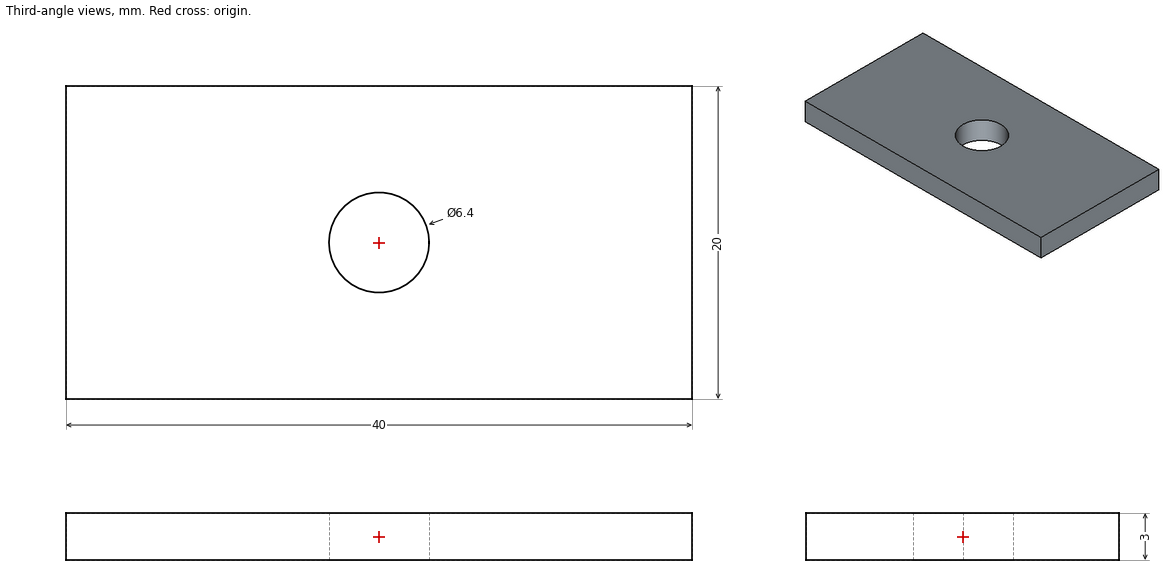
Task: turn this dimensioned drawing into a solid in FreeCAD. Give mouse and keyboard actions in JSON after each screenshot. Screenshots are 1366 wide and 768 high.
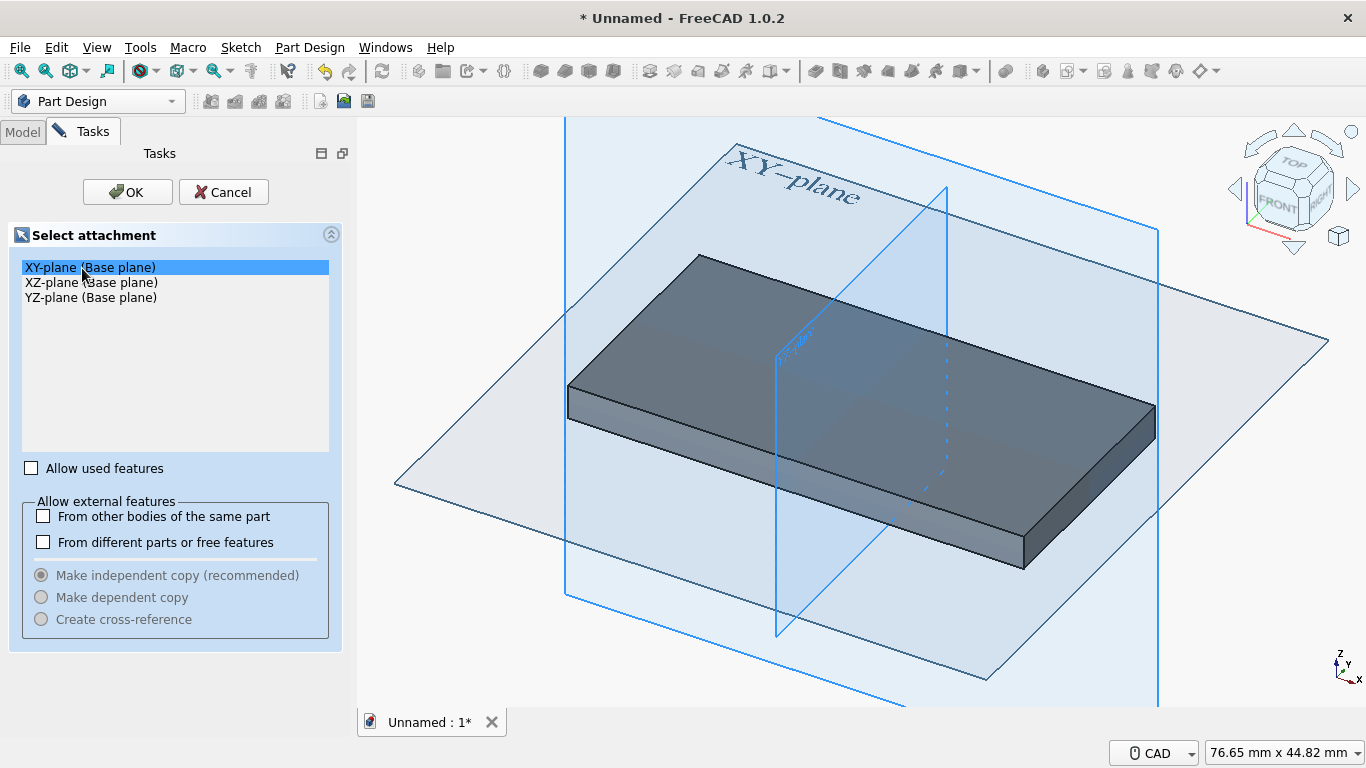
{"action": "left_click", "coordinate": [128, 192]}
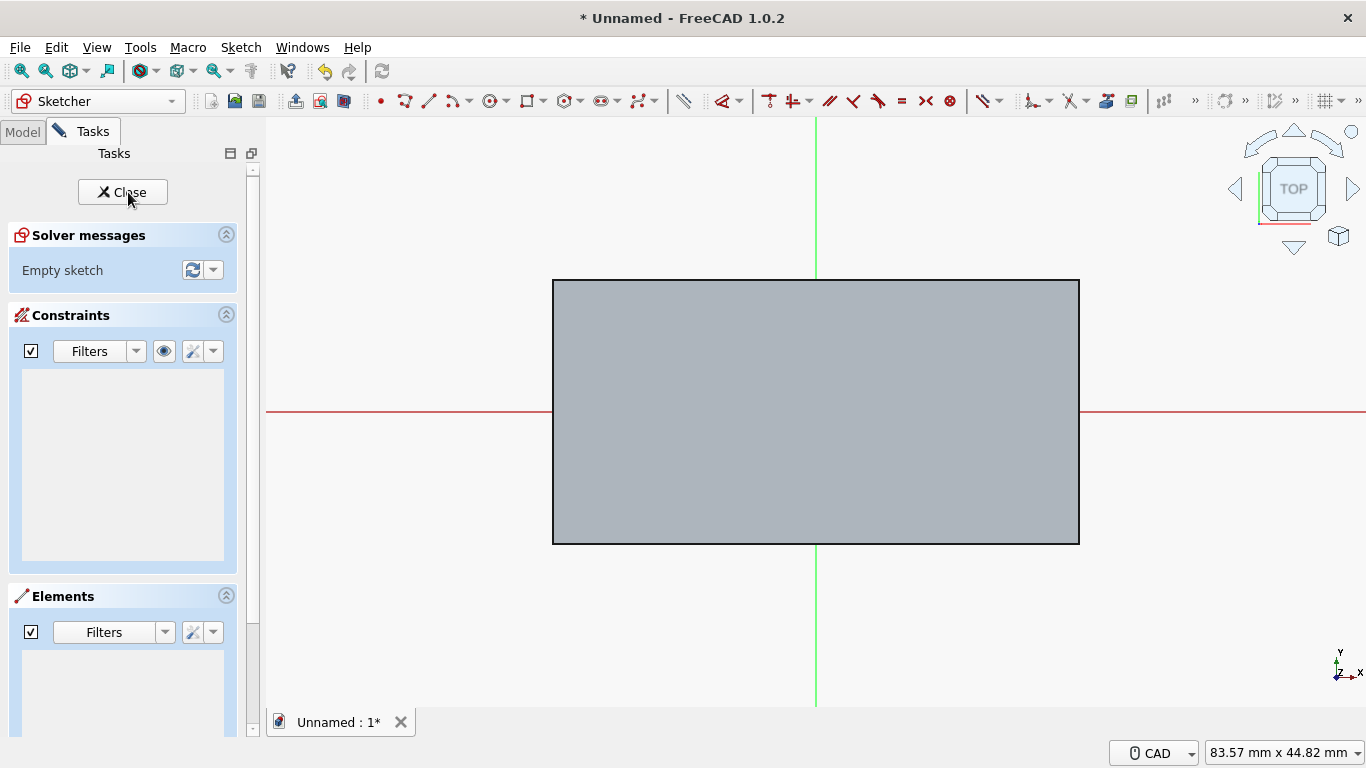
{"action": "key", "text": "q s"}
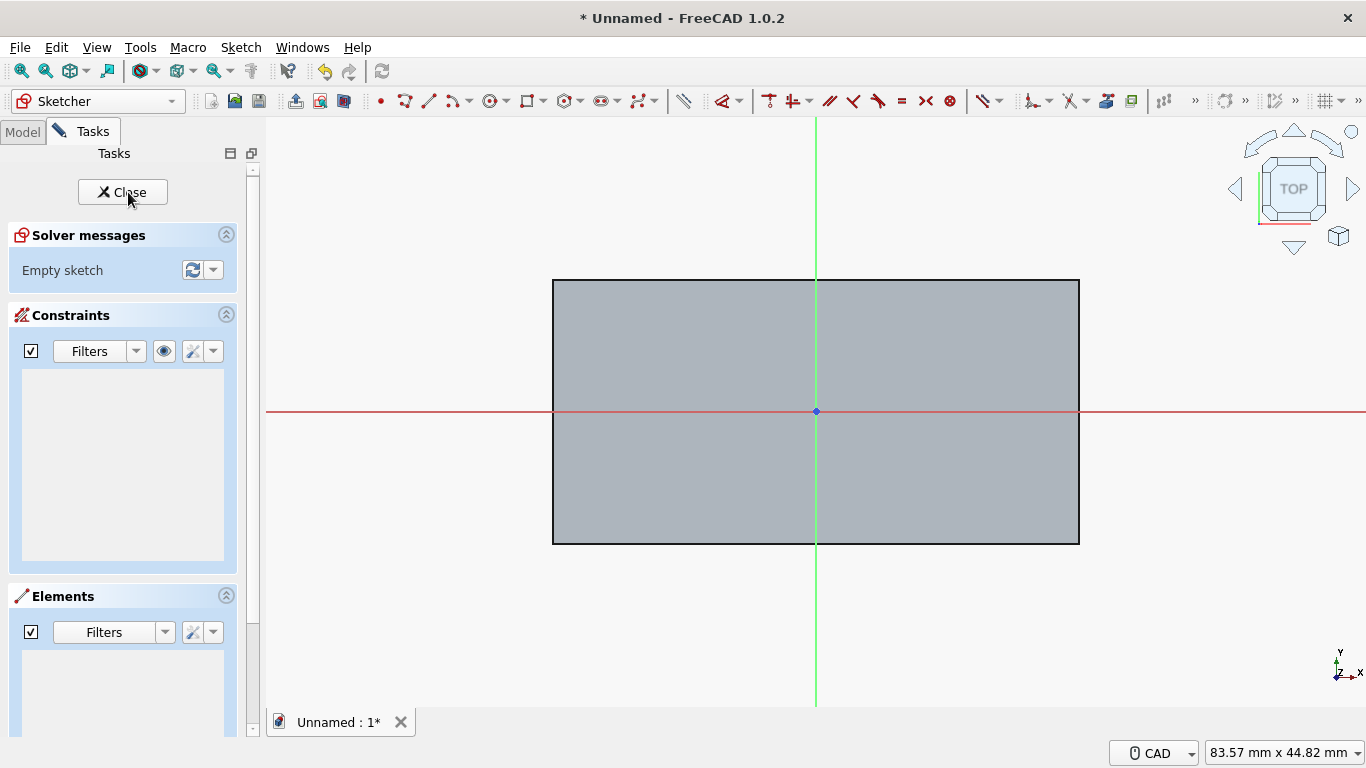
{"action": "scroll", "coordinate": [838, 412], "scroll_direction": "up", "scroll_amount": 7}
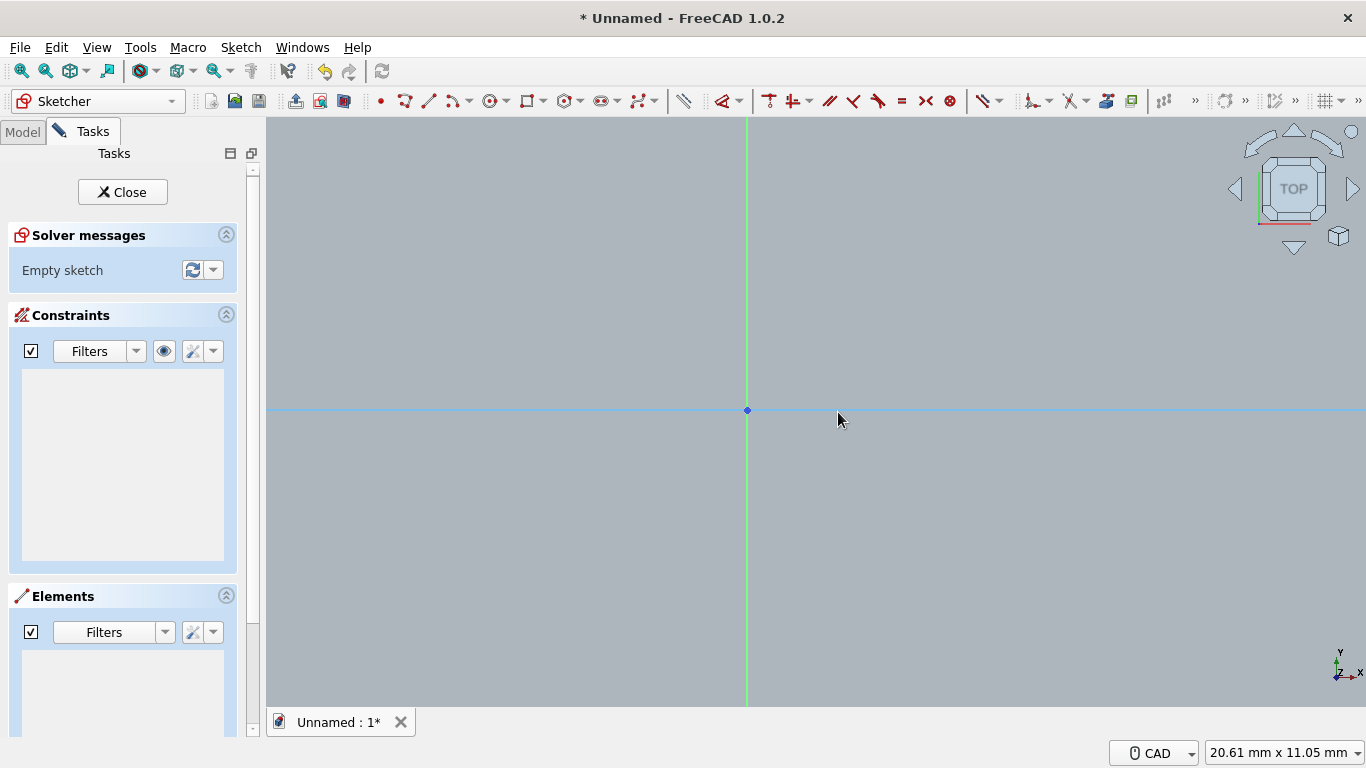
{"action": "left_click", "coordinate": [490, 102]}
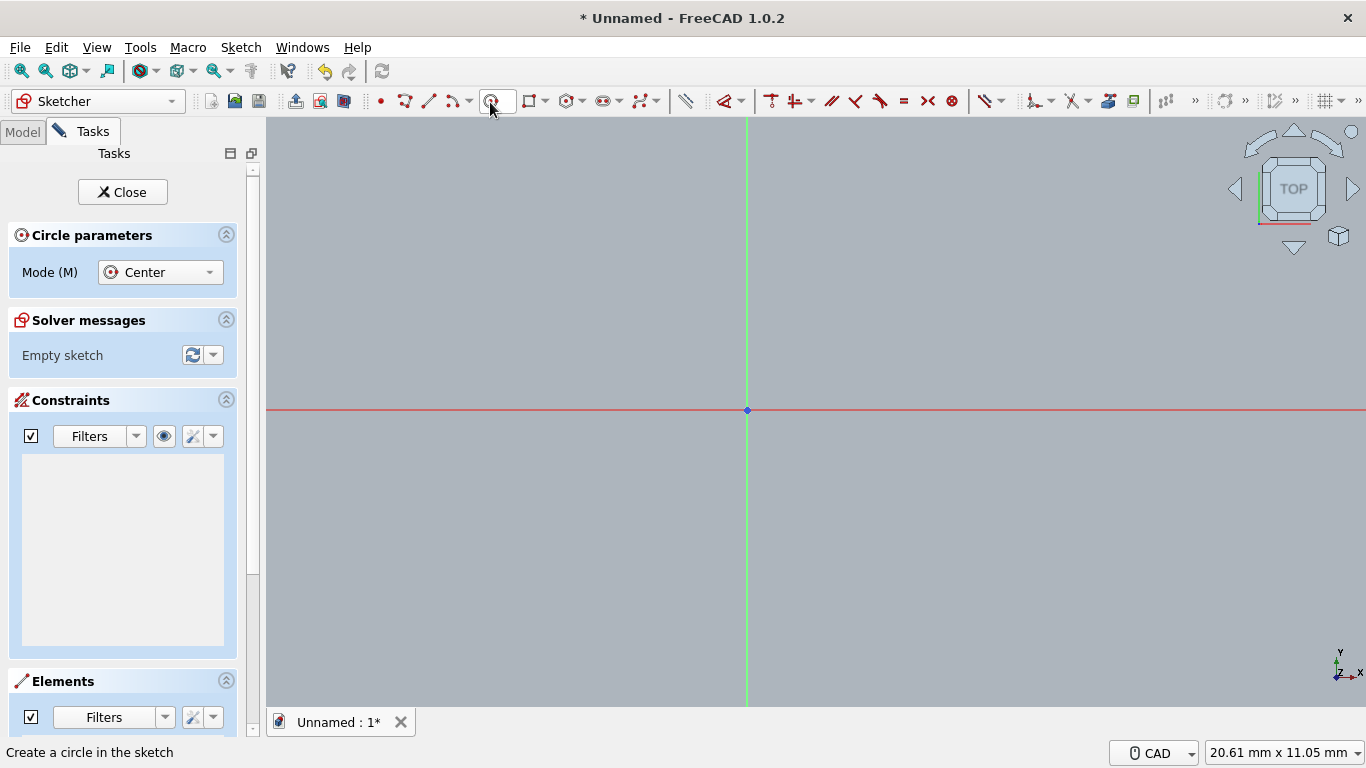
{"action": "left_click", "coordinate": [747, 410]}
{"action": "left_click", "coordinate": [868, 290]}
{"action": "key", "text": "Escape"}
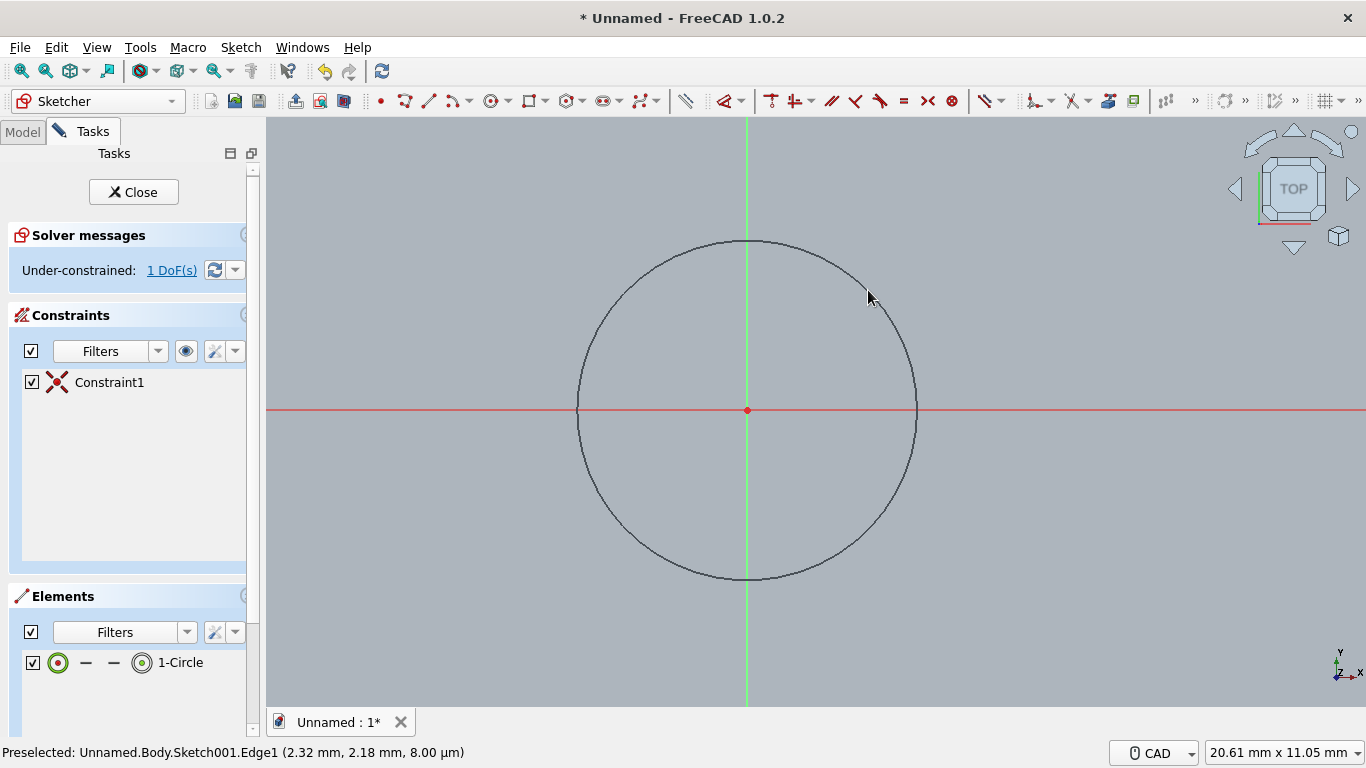
{"action": "left_click", "coordinate": [724, 102]}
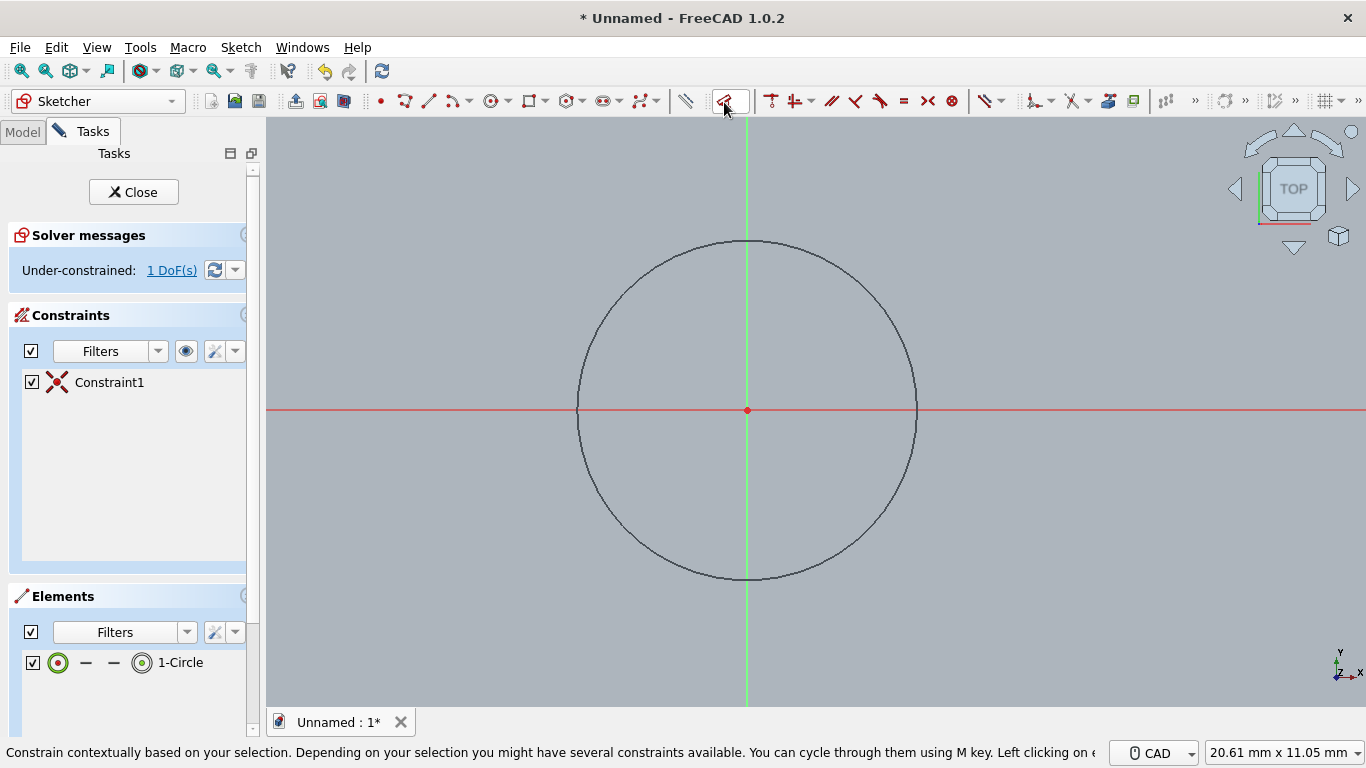
{"action": "left_click", "coordinate": [867, 290]}
{"action": "left_click", "coordinate": [890, 267]}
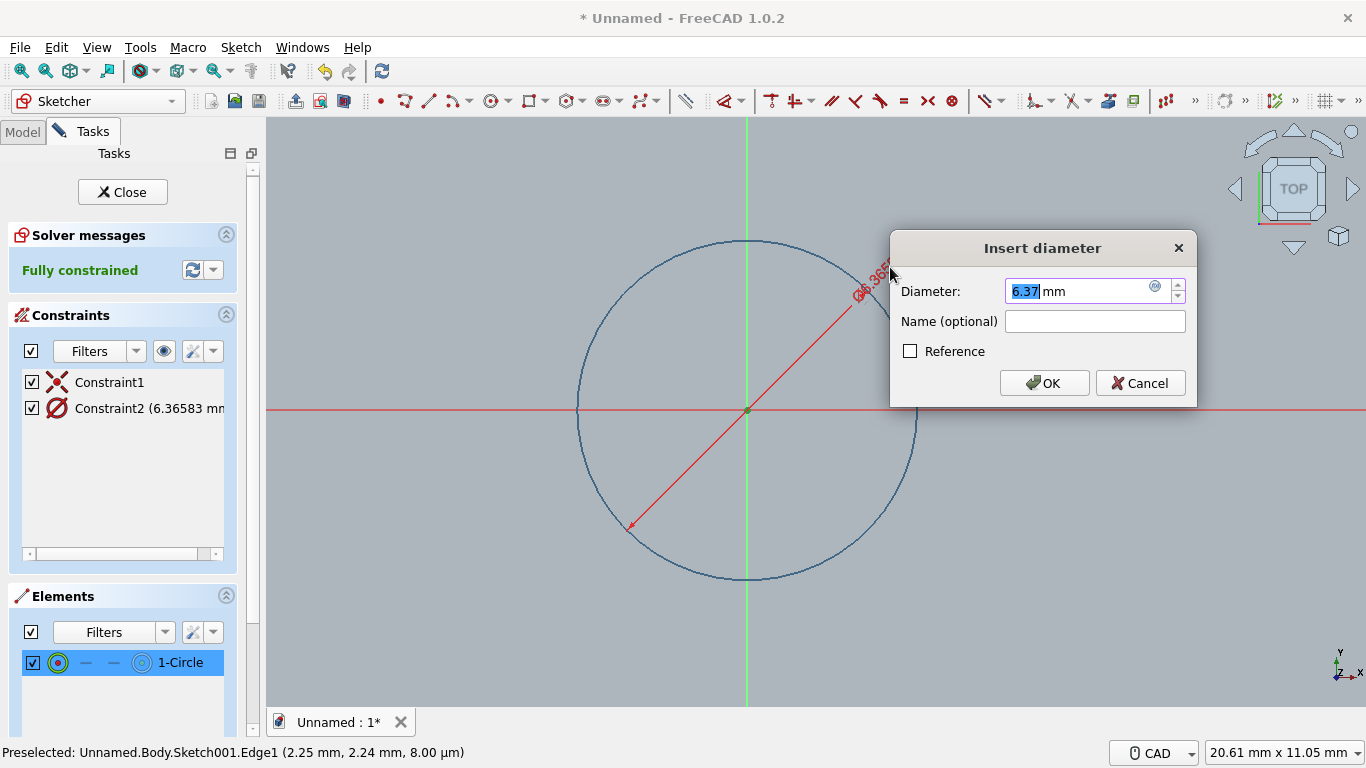
{"action": "type", "text": "6.4"}
{"action": "key", "text": "Return"}
{"action": "key", "text": "Escape"}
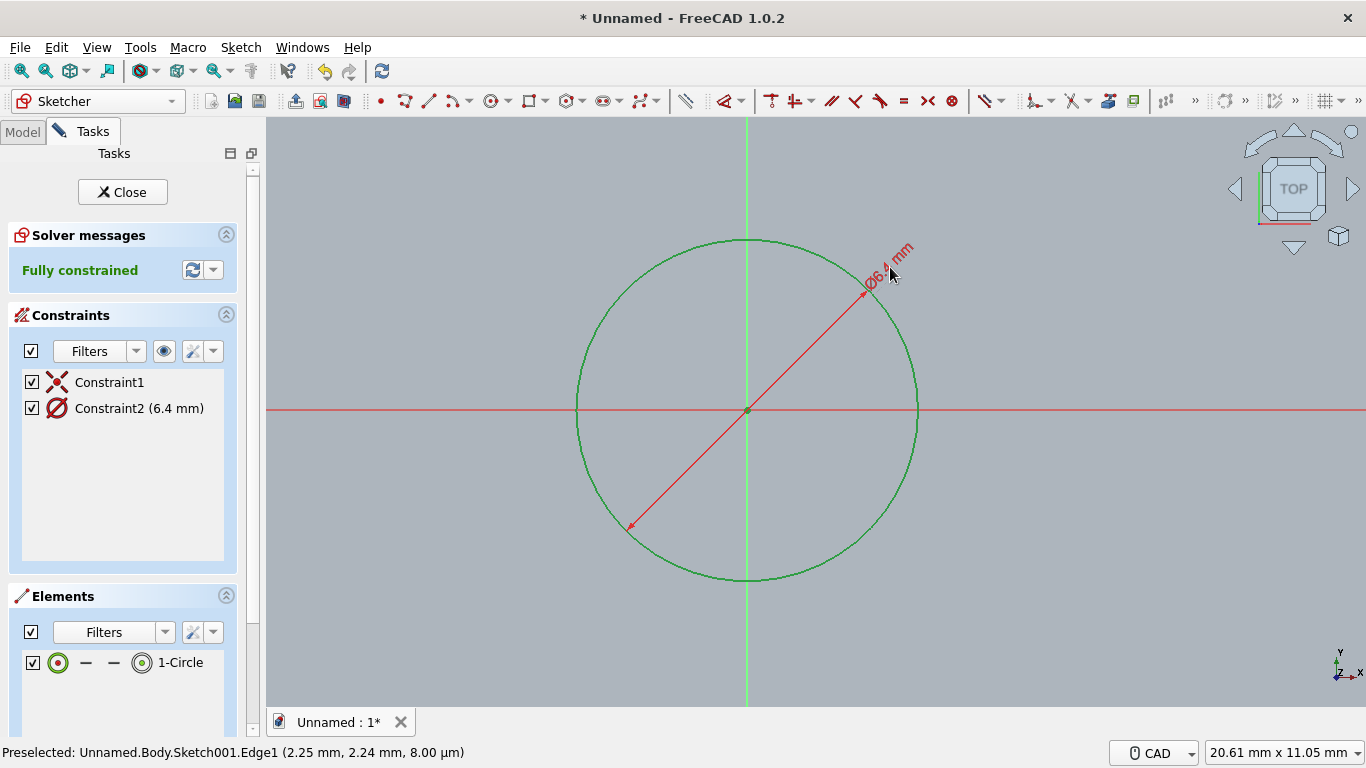
{"action": "left_click", "coordinate": [123, 192]}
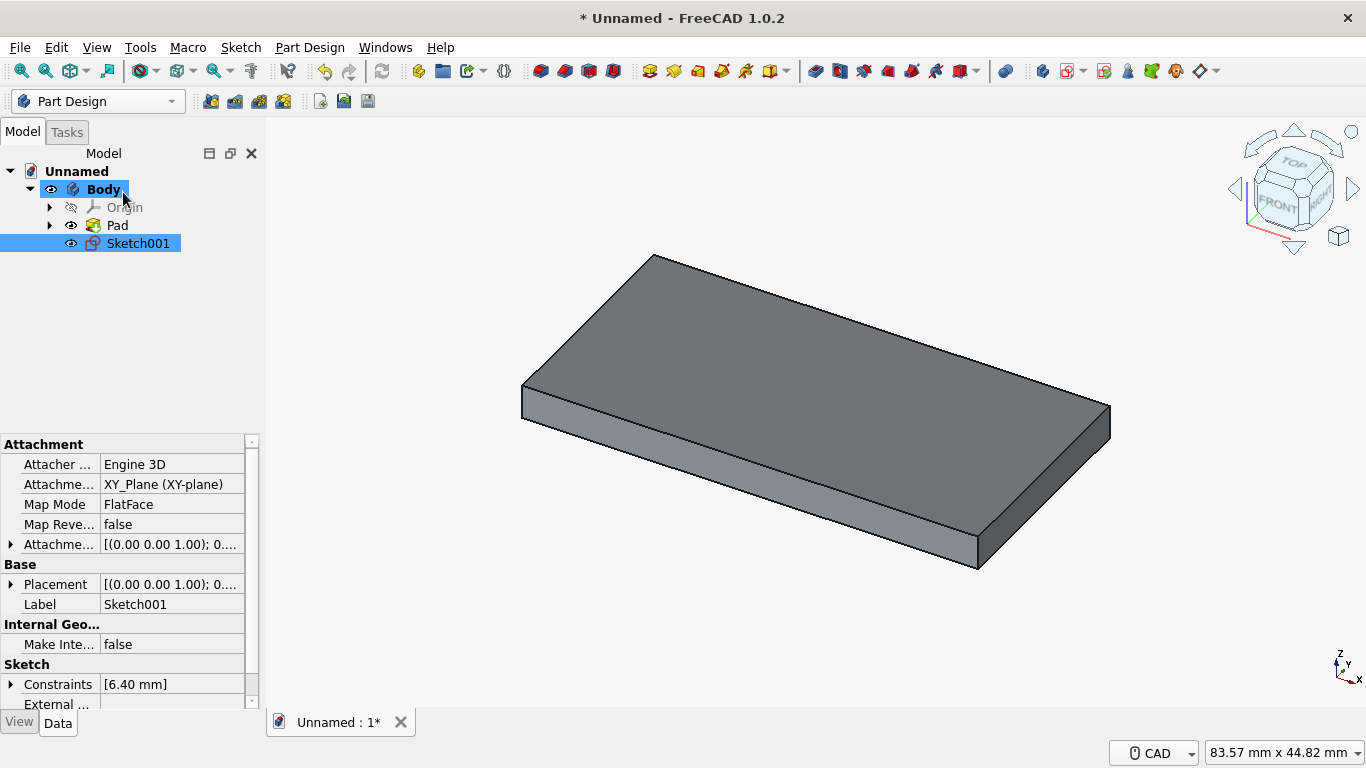
{"action": "left_click", "coordinate": [816, 72]}